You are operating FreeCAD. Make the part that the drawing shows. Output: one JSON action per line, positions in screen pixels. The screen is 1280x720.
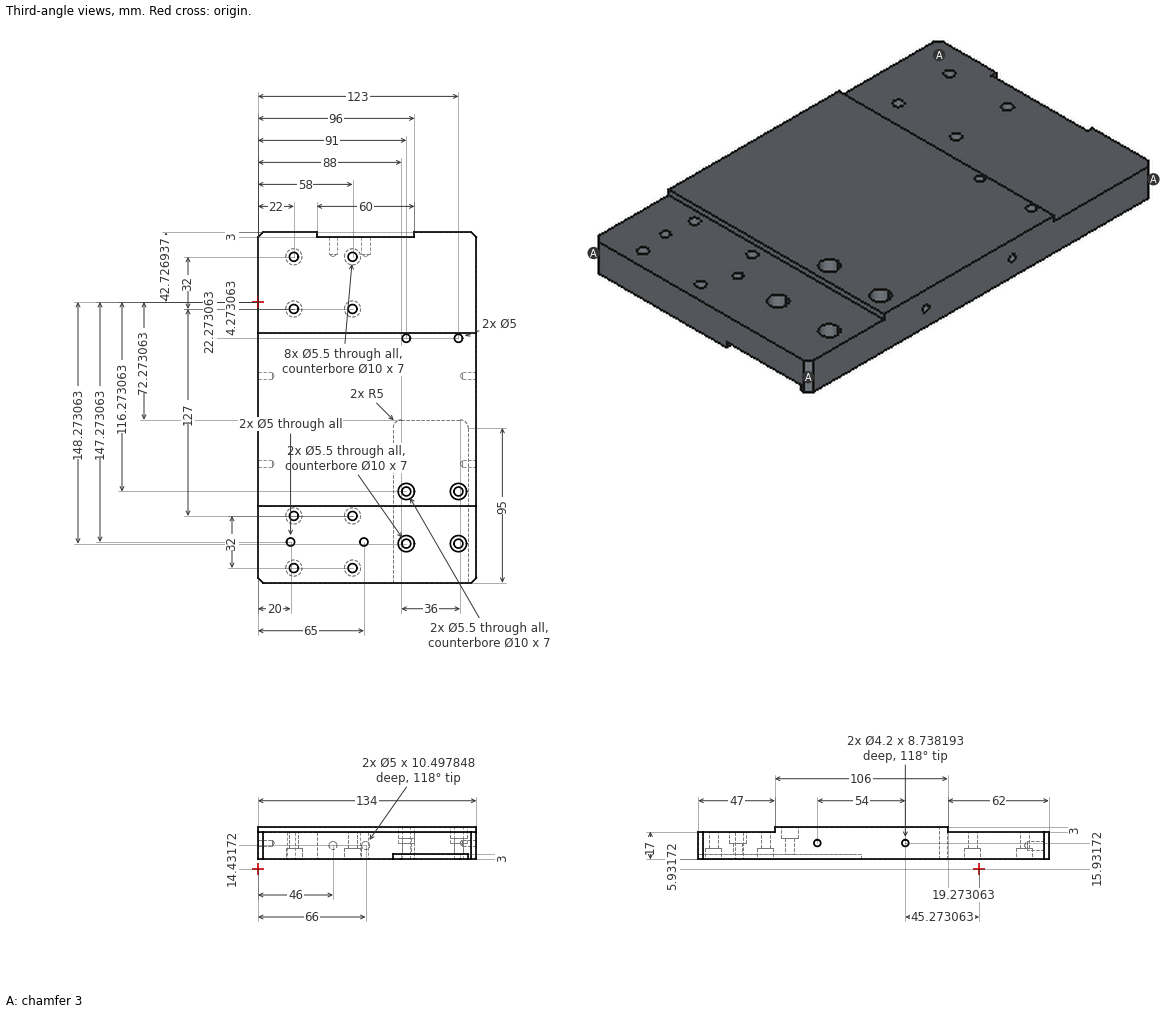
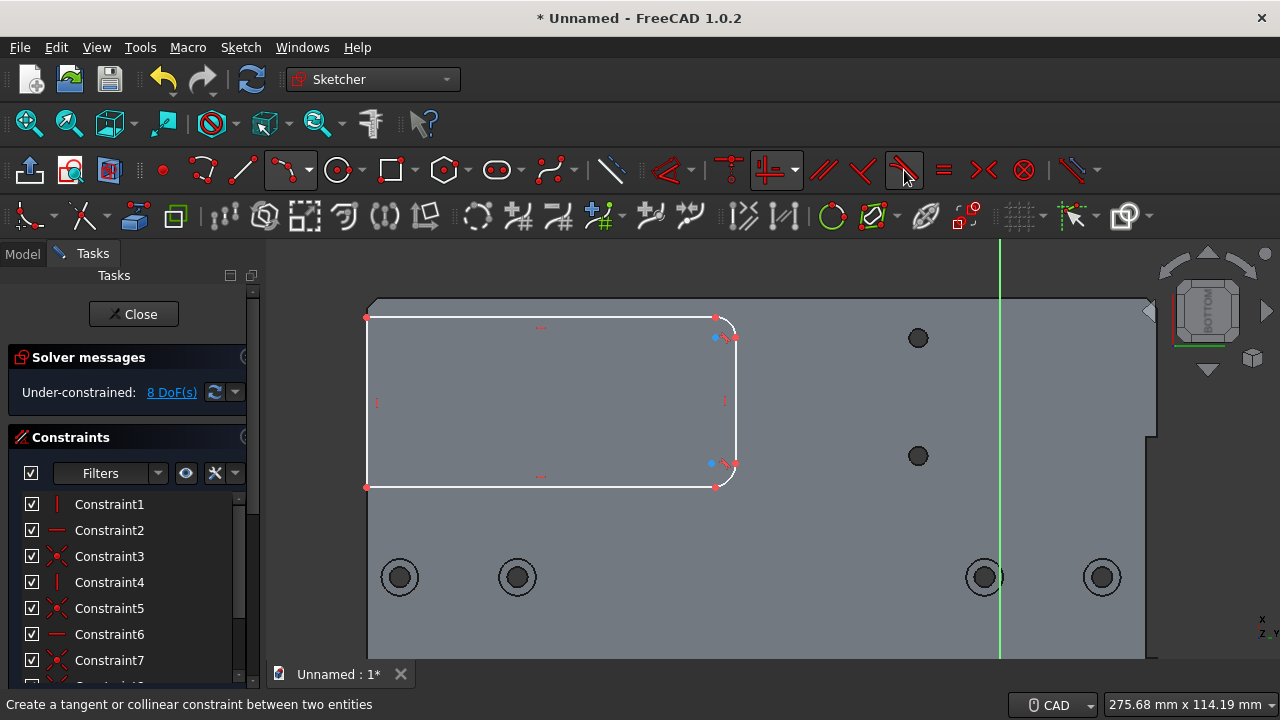
{"action": "left_click", "coordinate": [611, 317]}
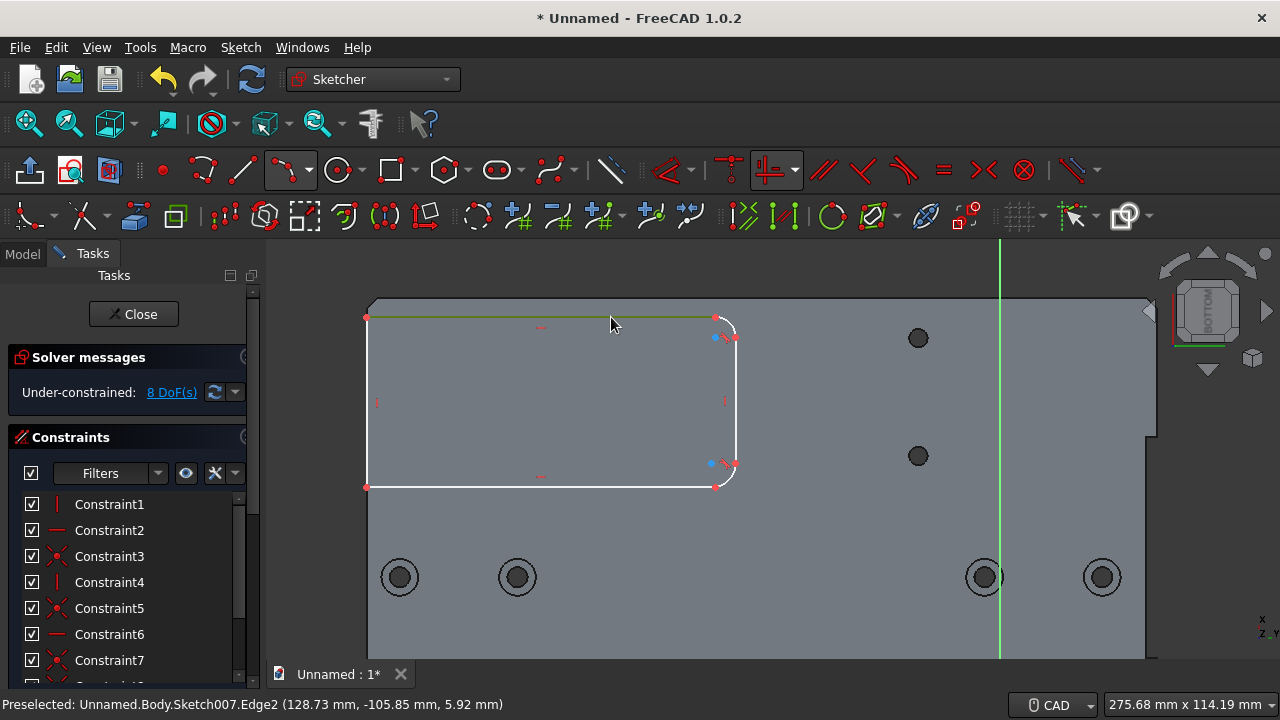
{"action": "scroll", "coordinate": [733, 328], "scroll_direction": "up", "scroll_amount": 2}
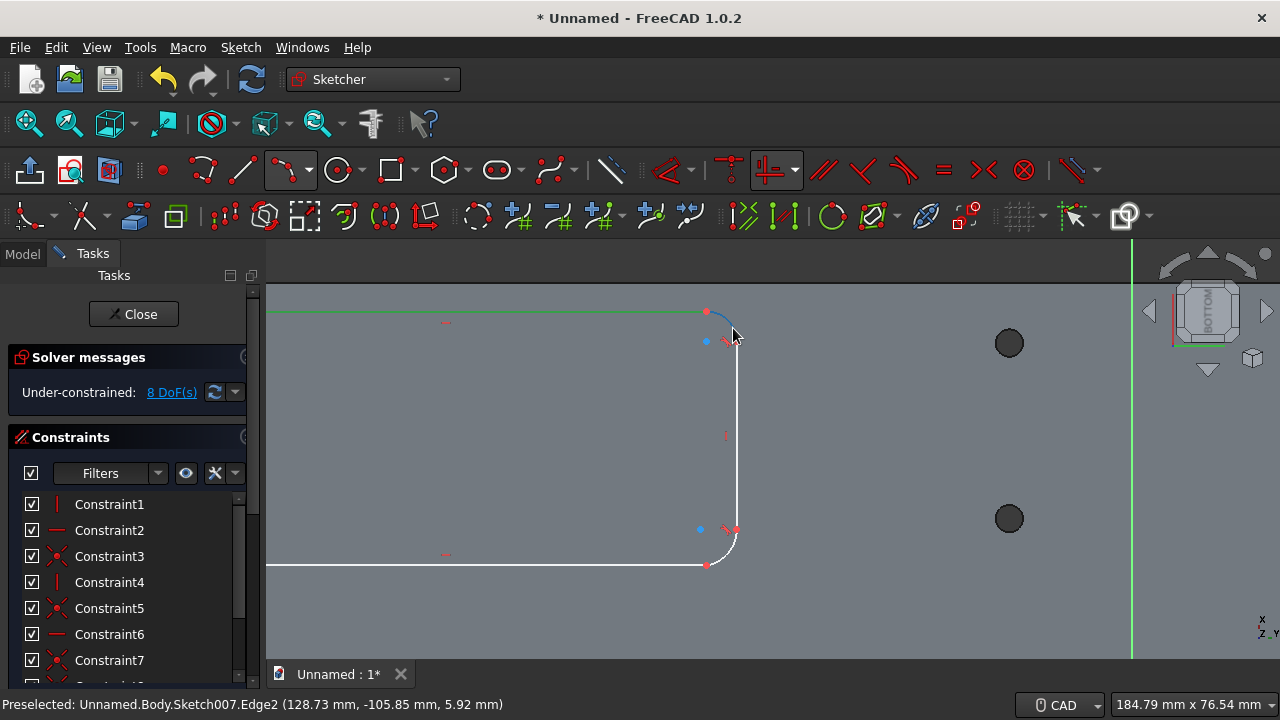
{"action": "left_click", "coordinate": [733, 328]}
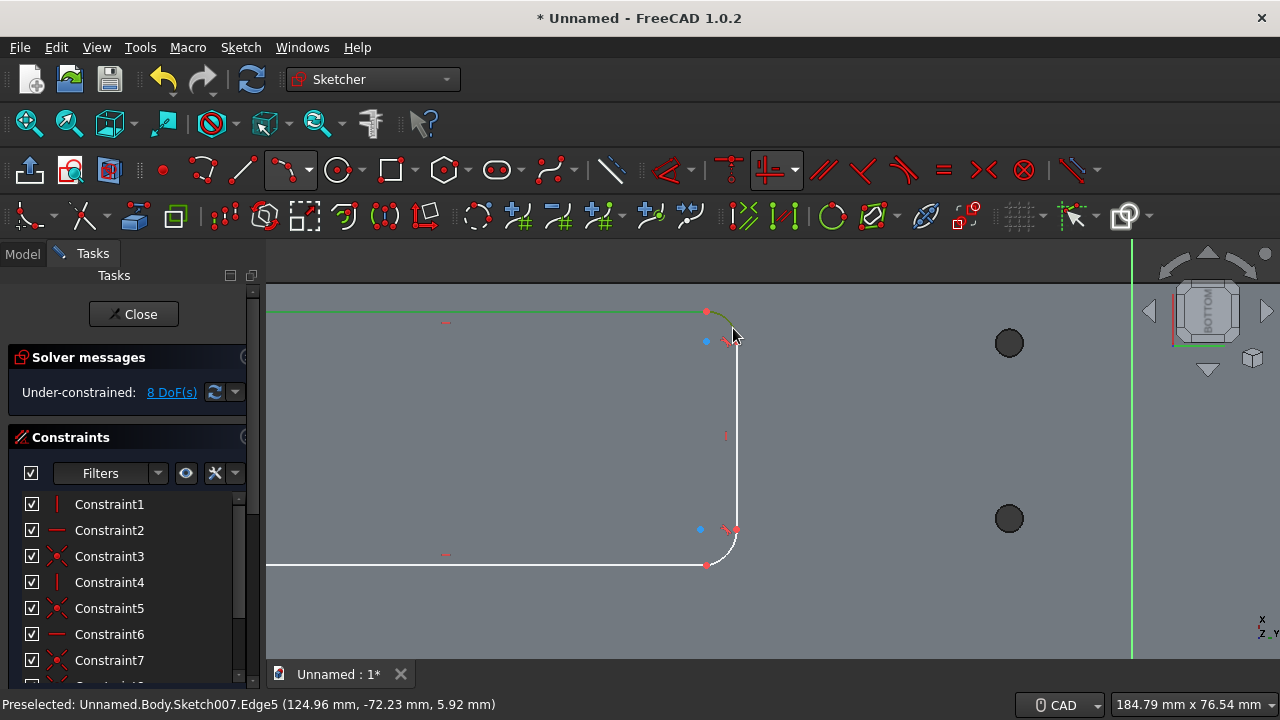
{"action": "left_click", "coordinate": [904, 170]}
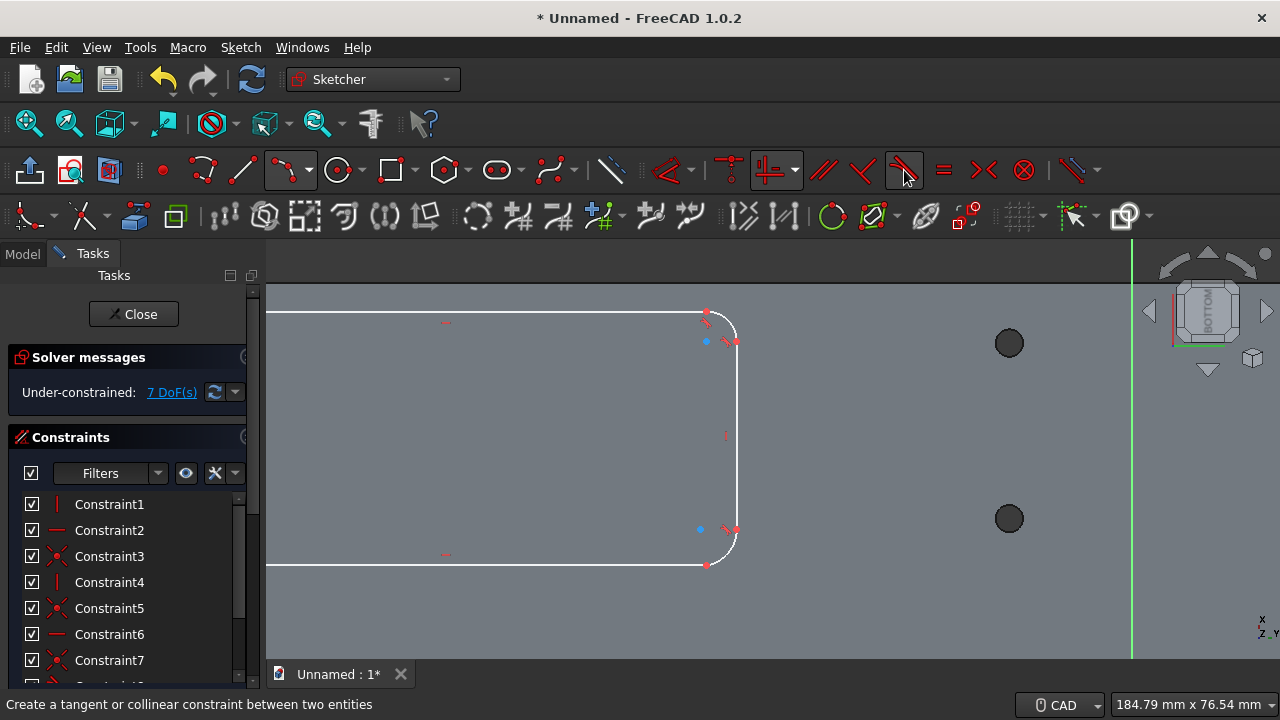
{"action": "left_click", "coordinate": [342, 565]}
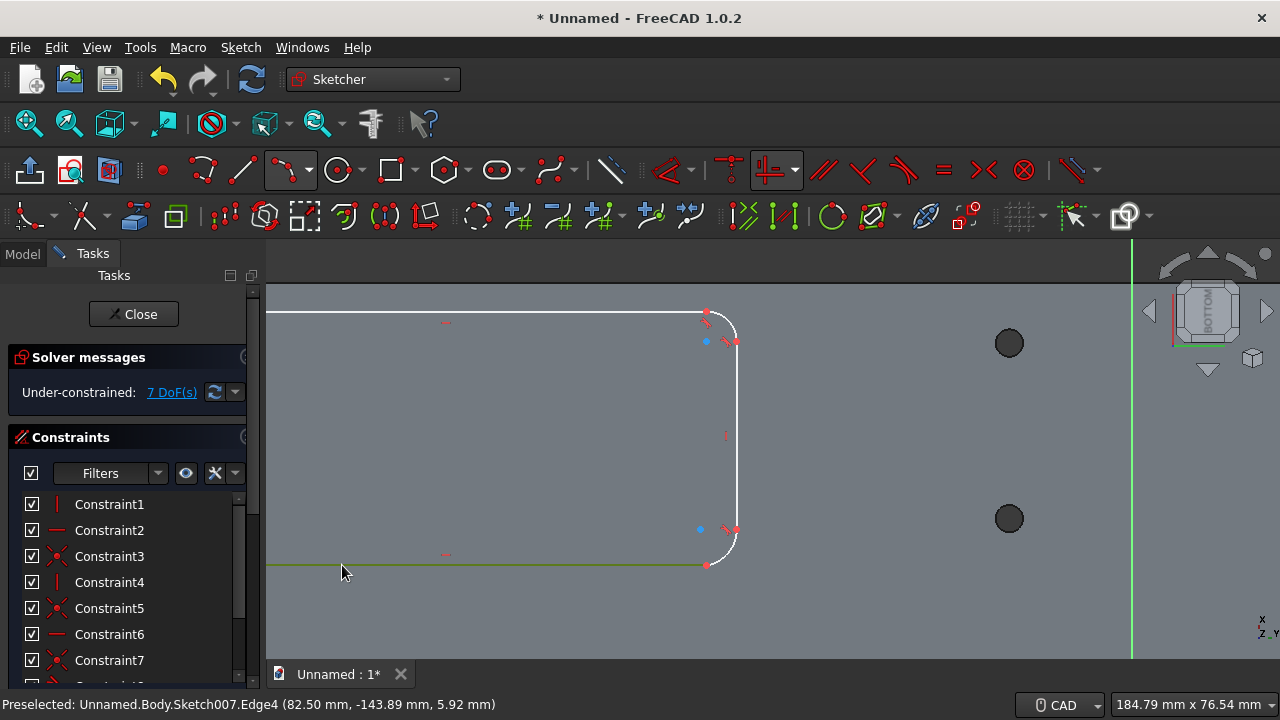
{"action": "left_click", "coordinate": [721, 560]}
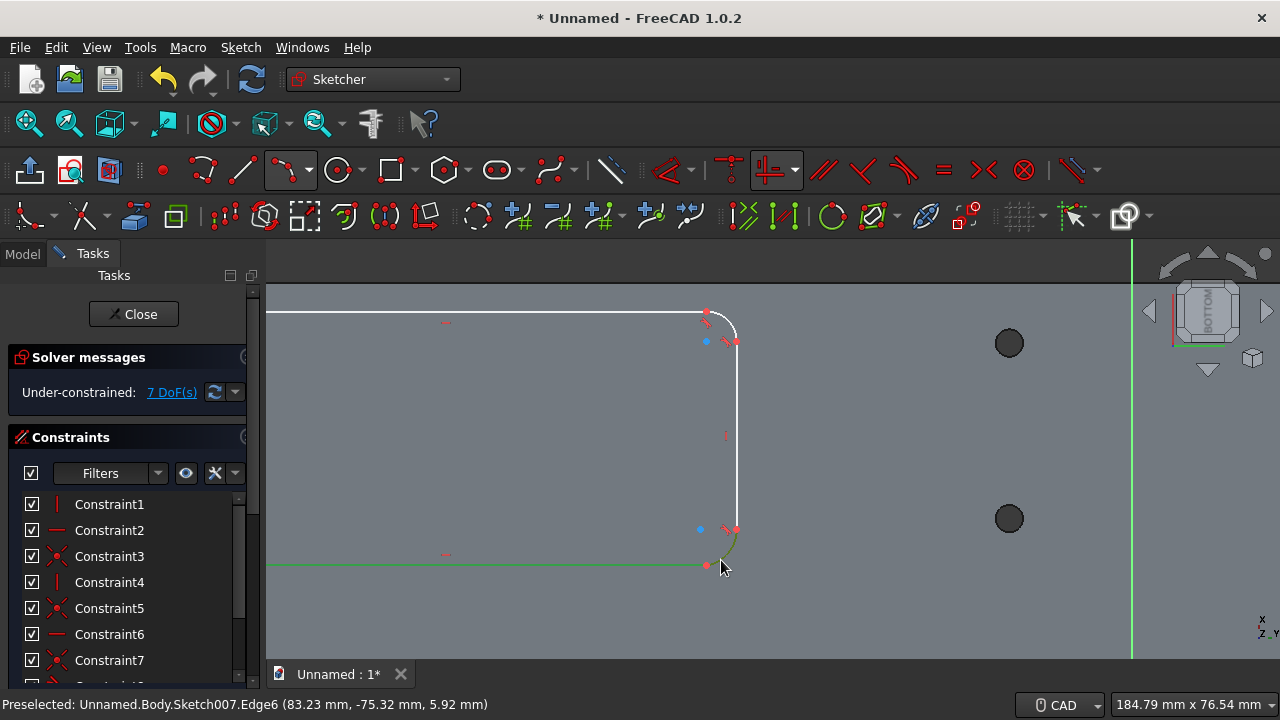
{"action": "left_click", "coordinate": [904, 170]}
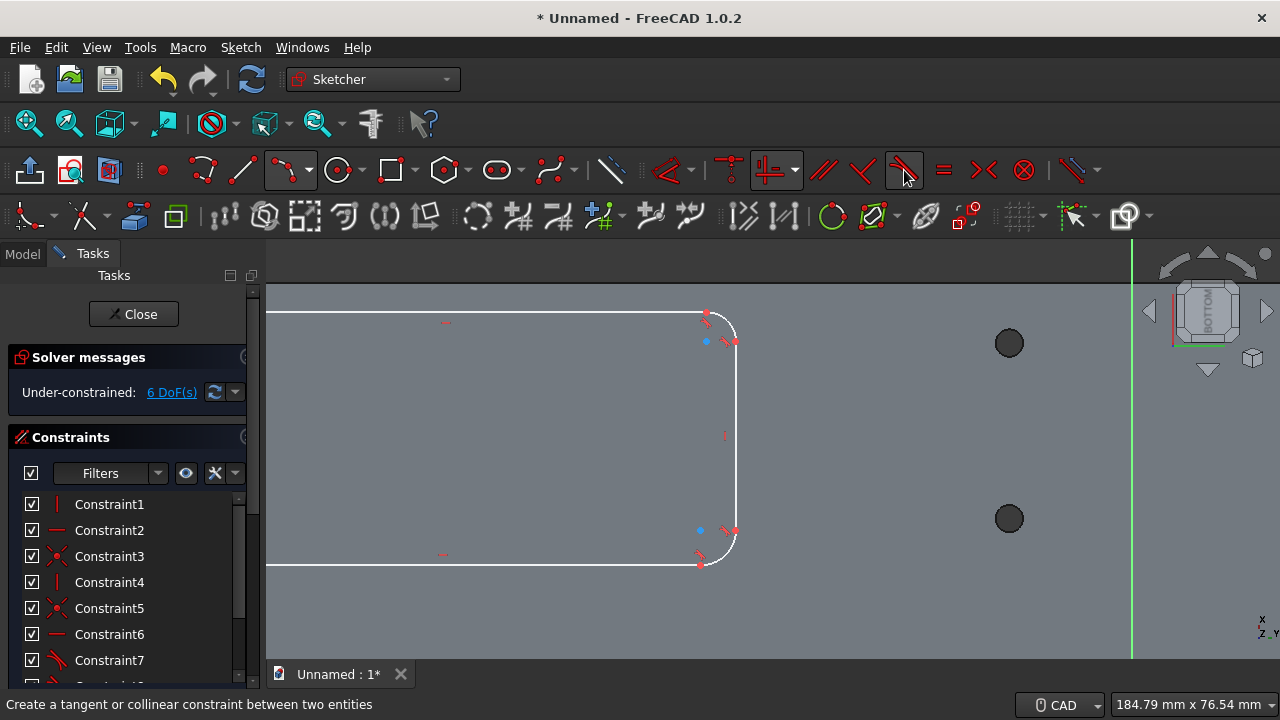
{"action": "left_click", "coordinate": [733, 328]}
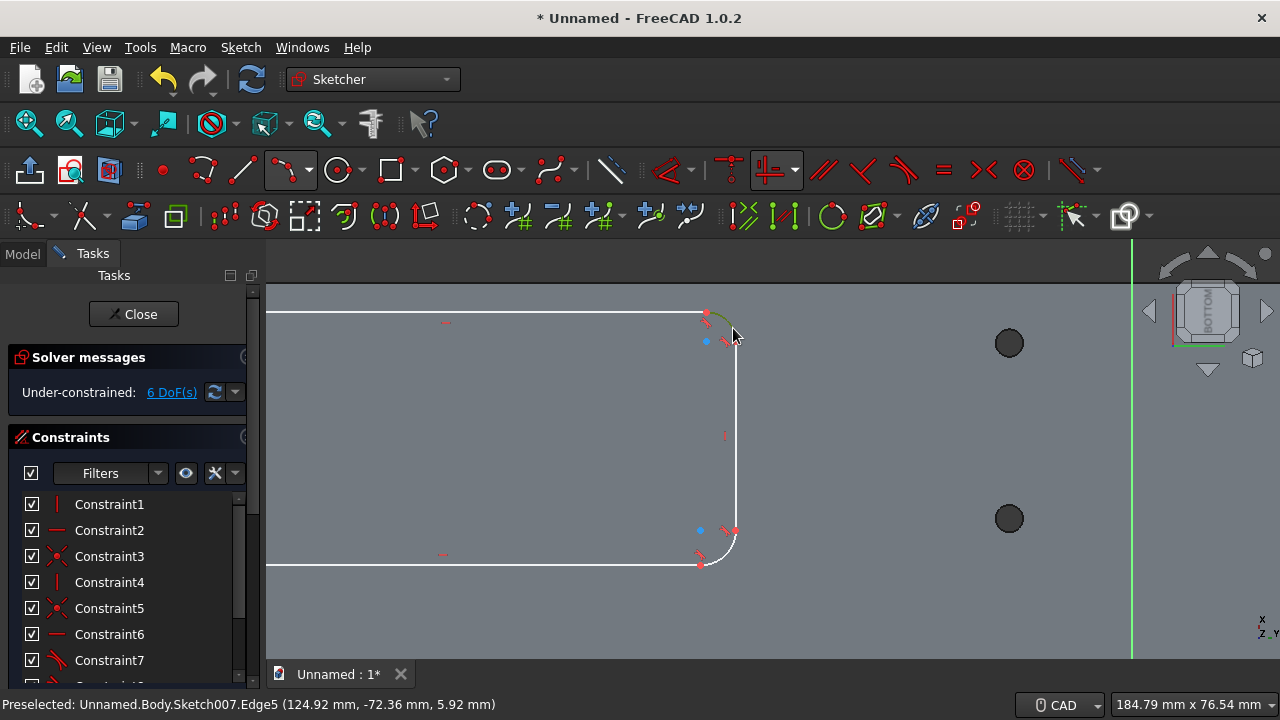
{"action": "left_click", "coordinate": [717, 561]}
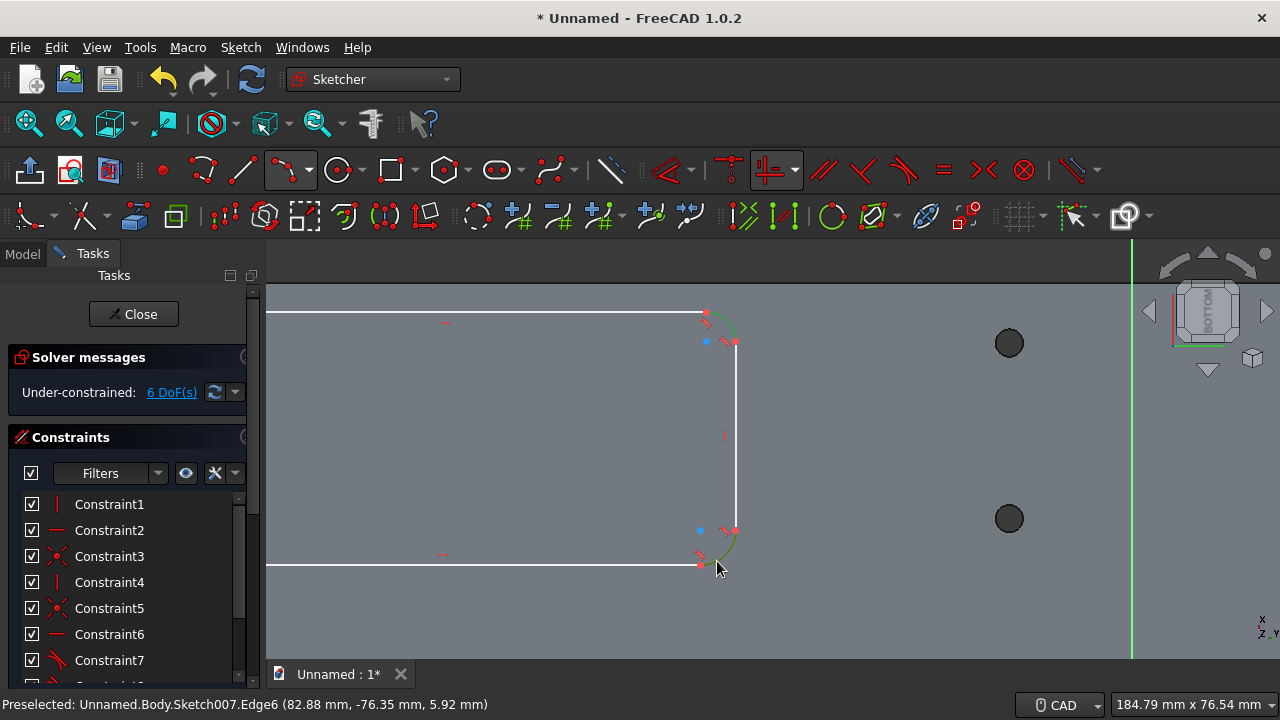
{"action": "left_click", "coordinate": [944, 170]}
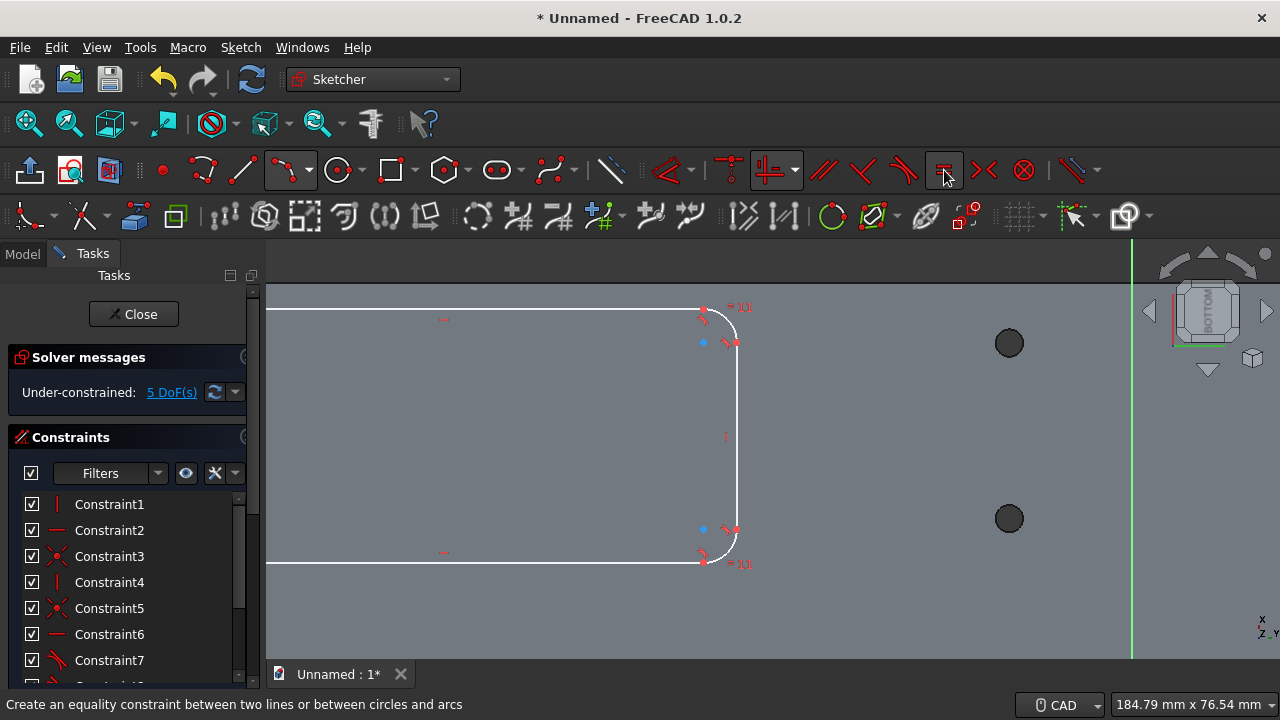
{"action": "left_click", "coordinate": [666, 170]}